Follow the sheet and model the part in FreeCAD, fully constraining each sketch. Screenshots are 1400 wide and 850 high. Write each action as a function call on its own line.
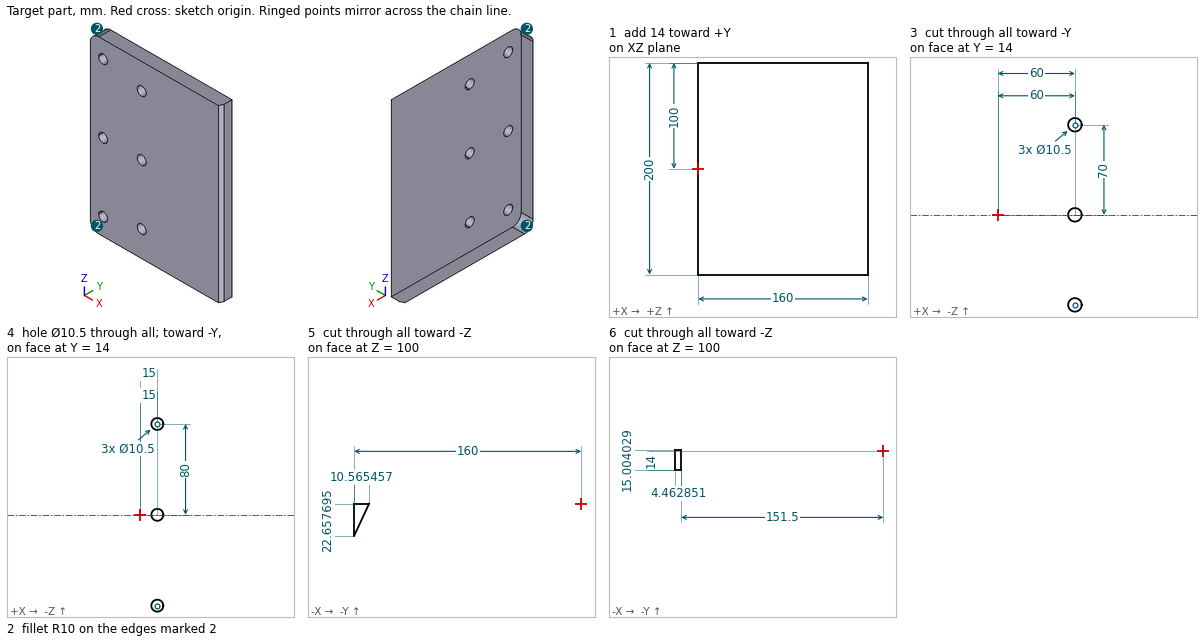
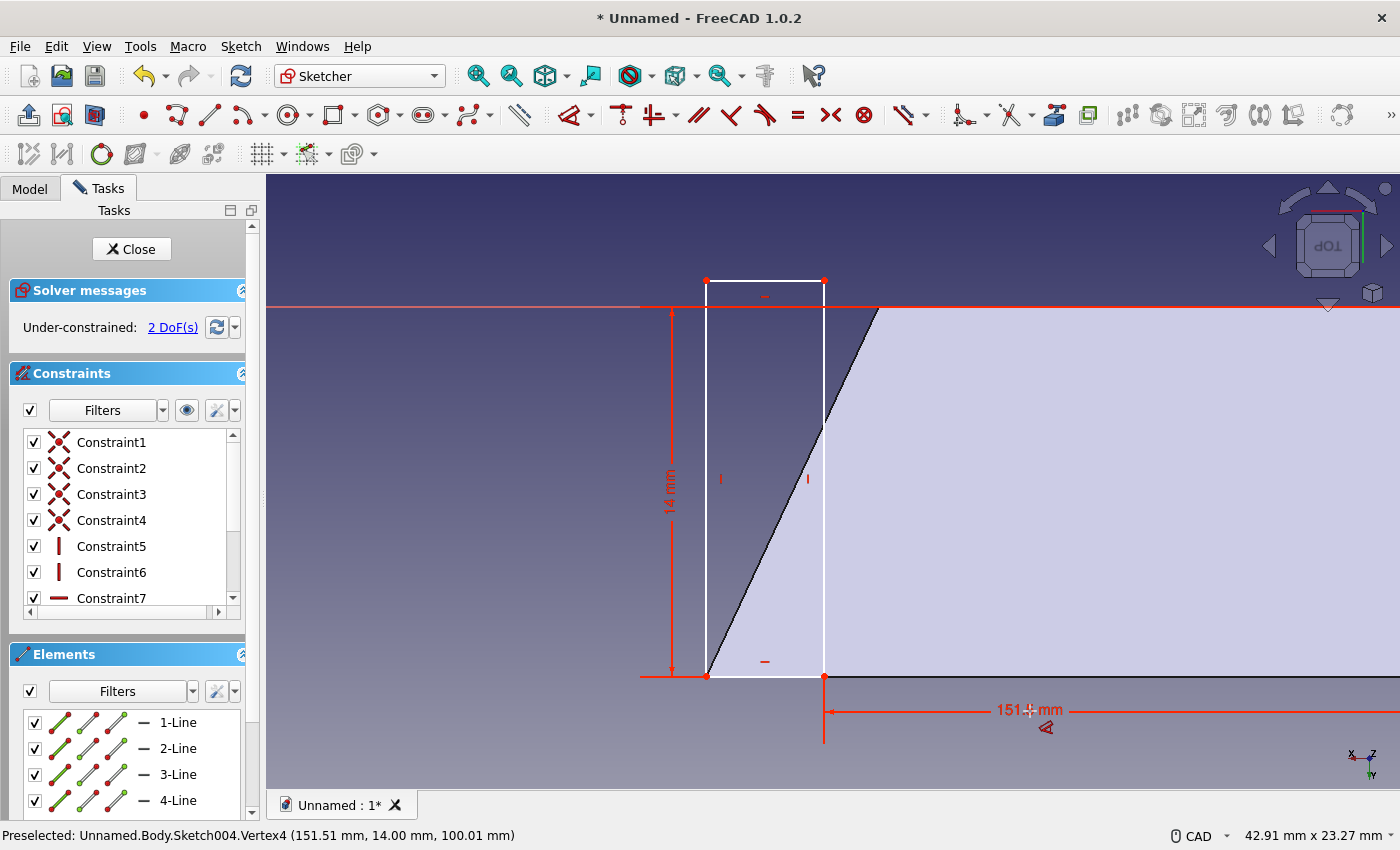
click(741, 677)
click(765, 711)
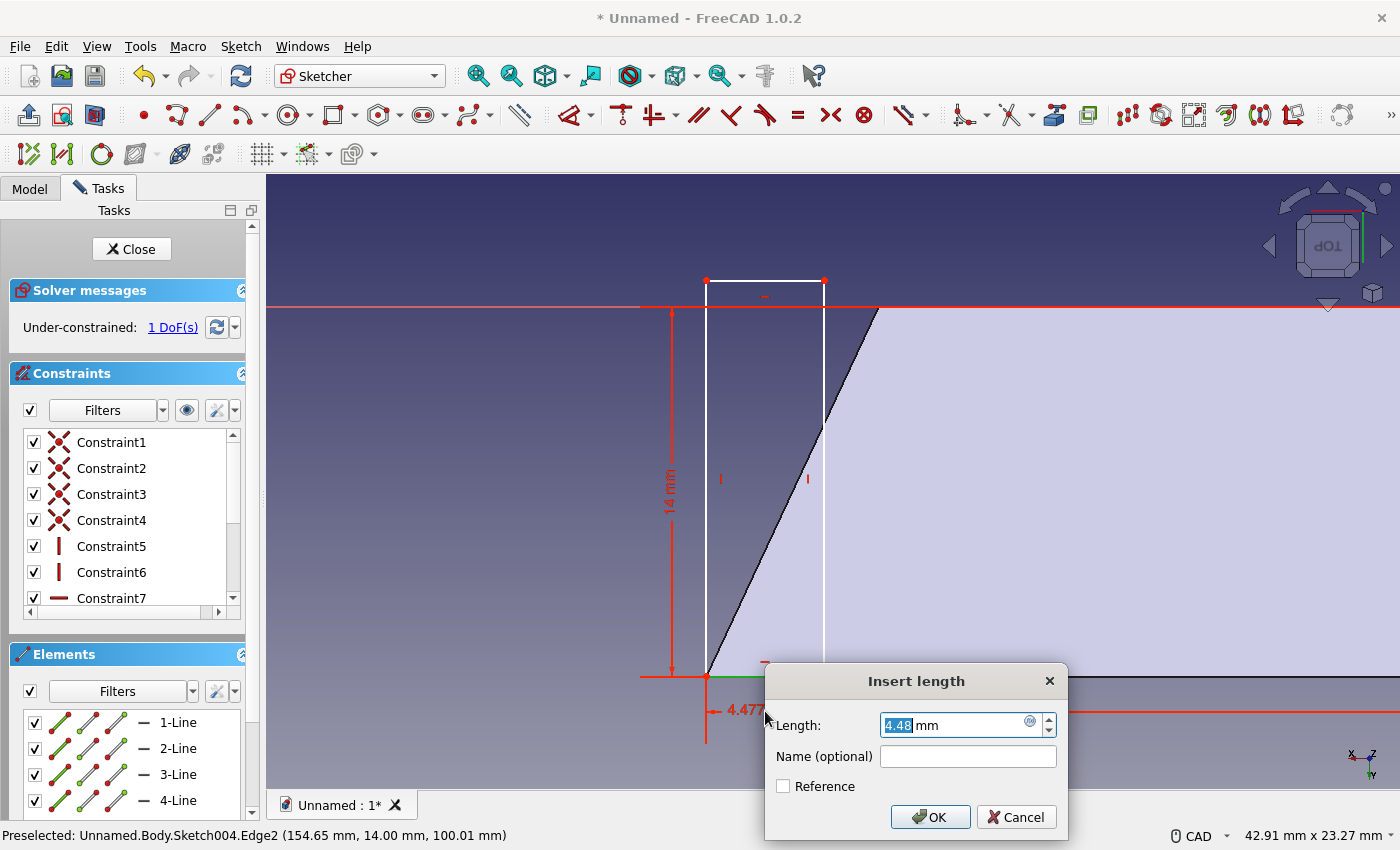
text(4.462851)
key(Return)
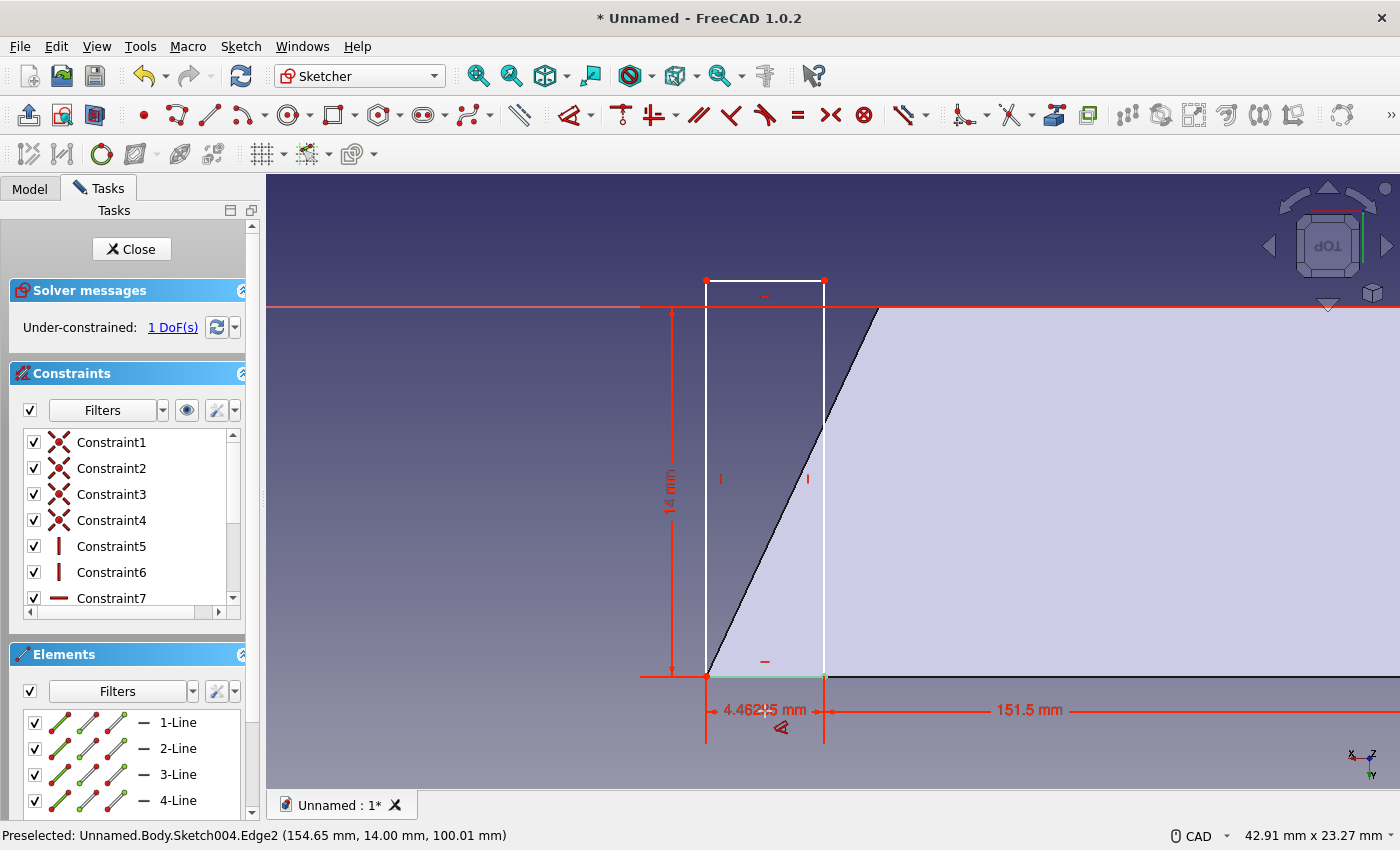
click(706, 400)
click(672, 388)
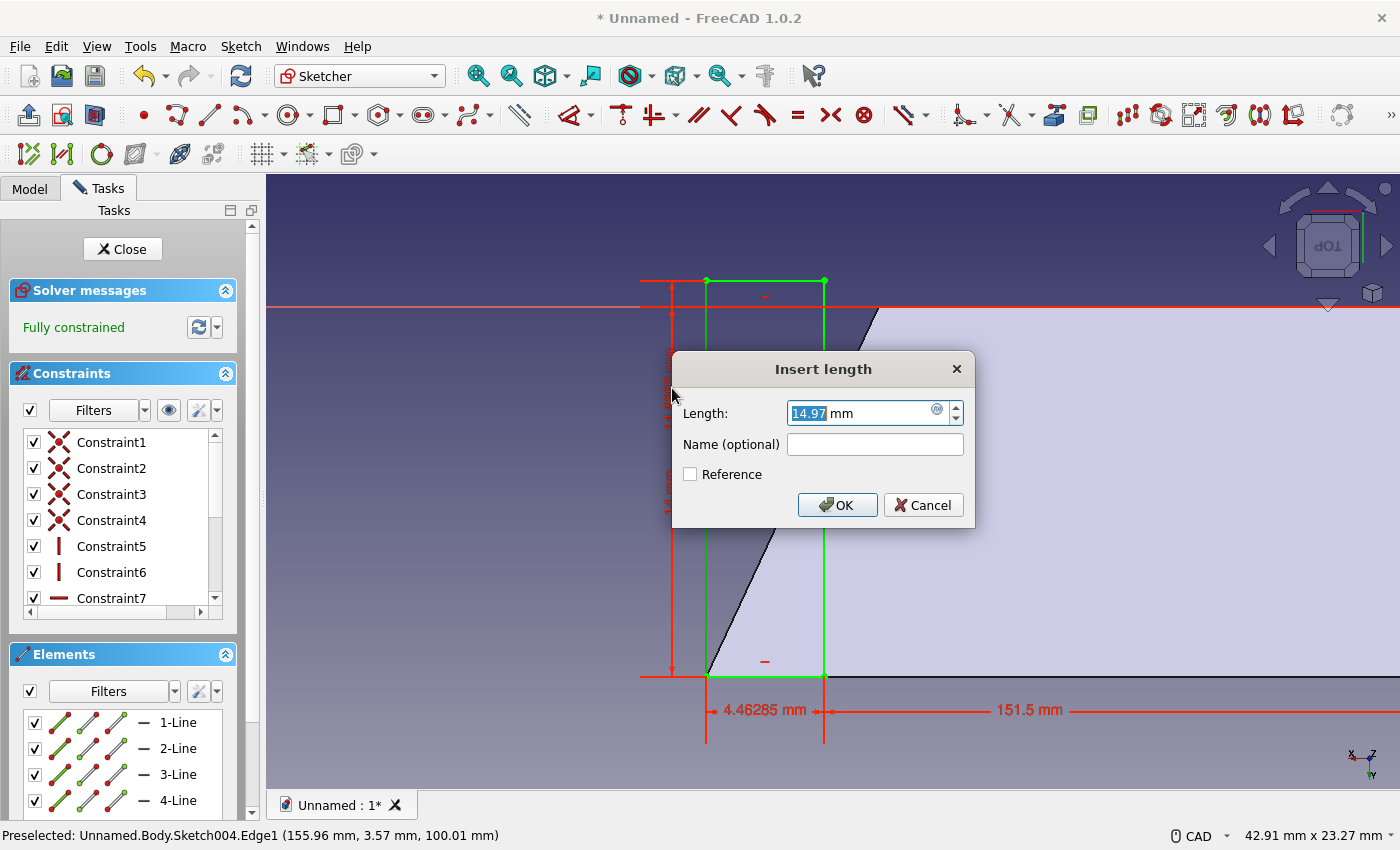
text(15.004029)
key(Return)
key(Escape)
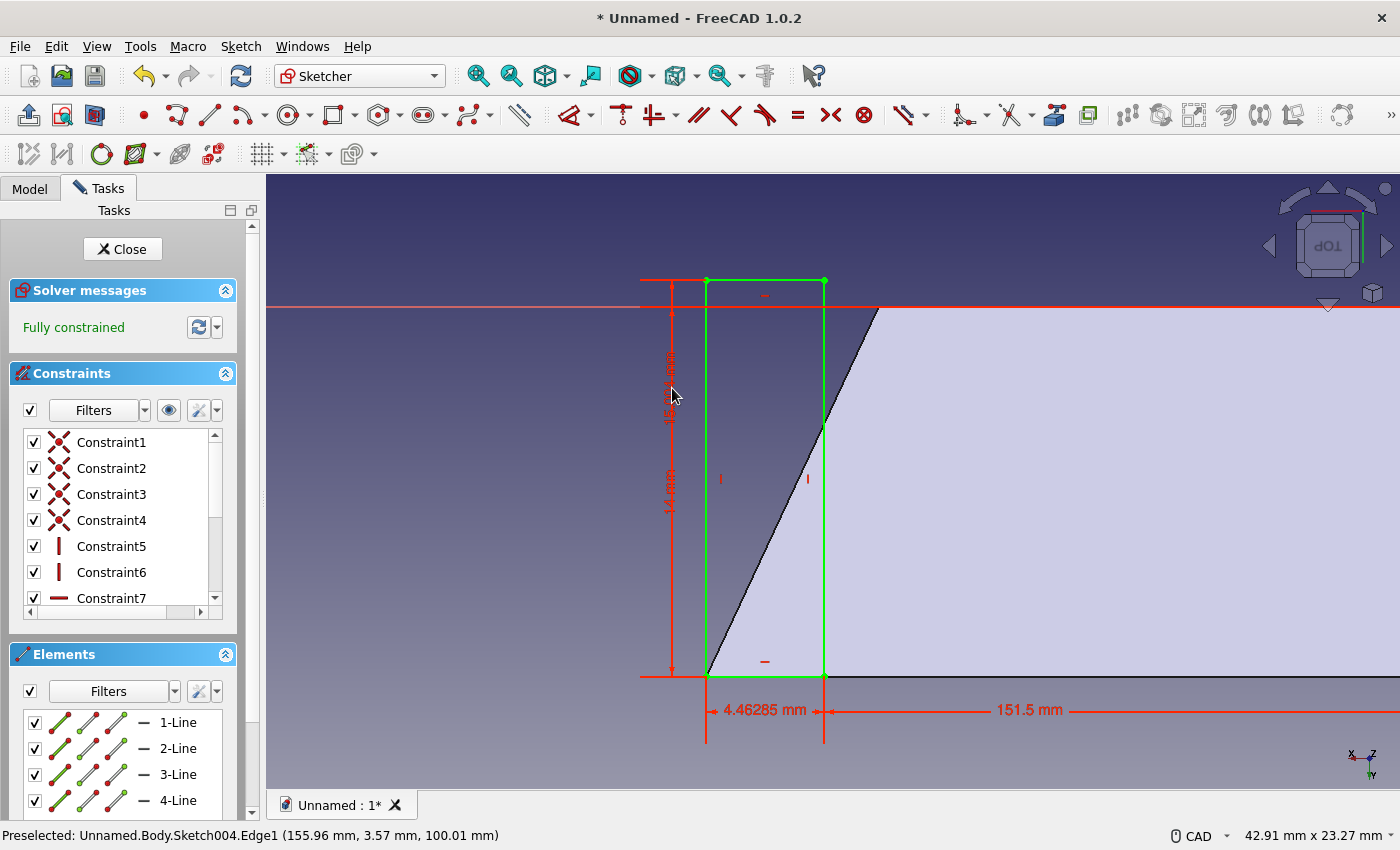
click(123, 249)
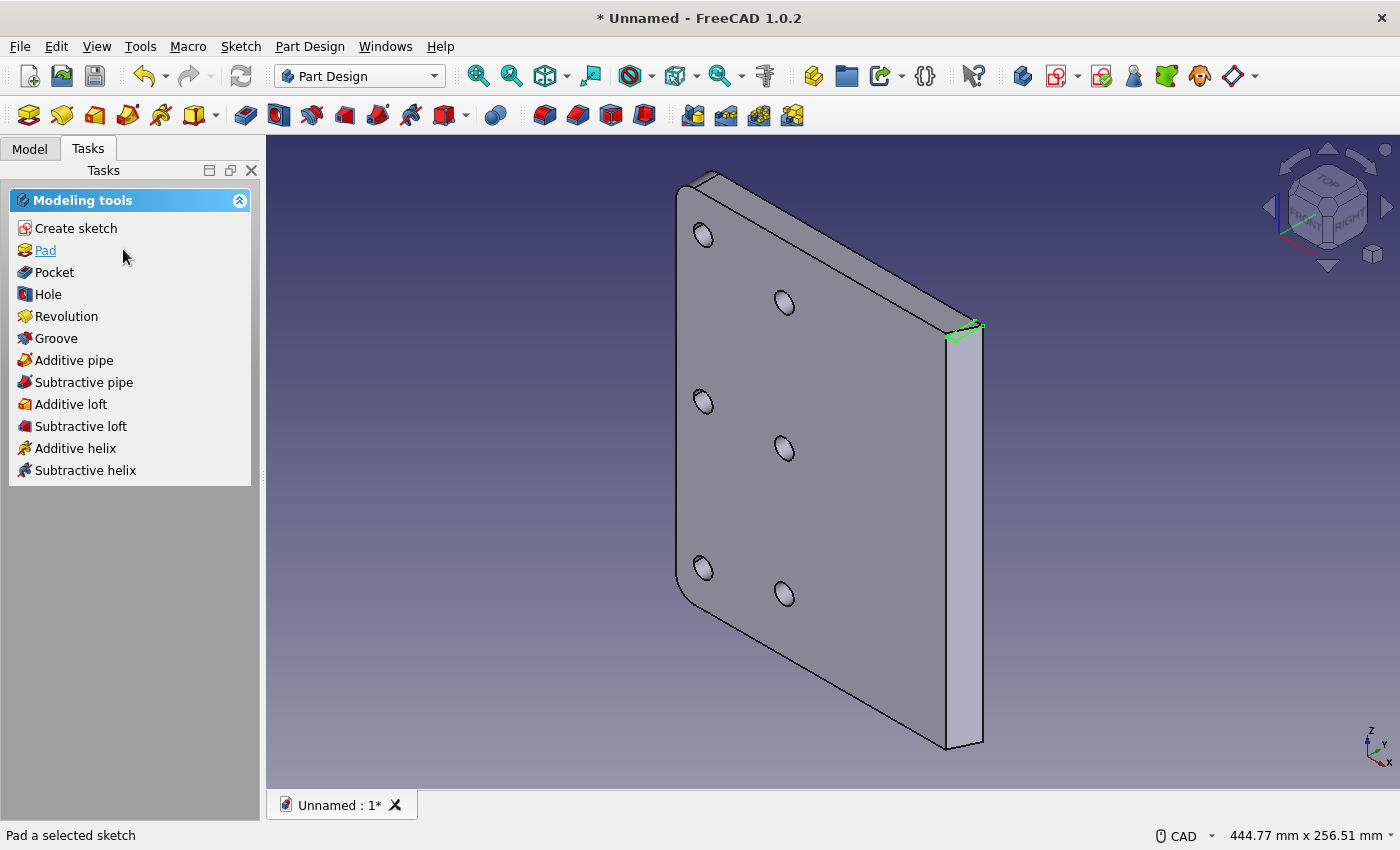
click(246, 116)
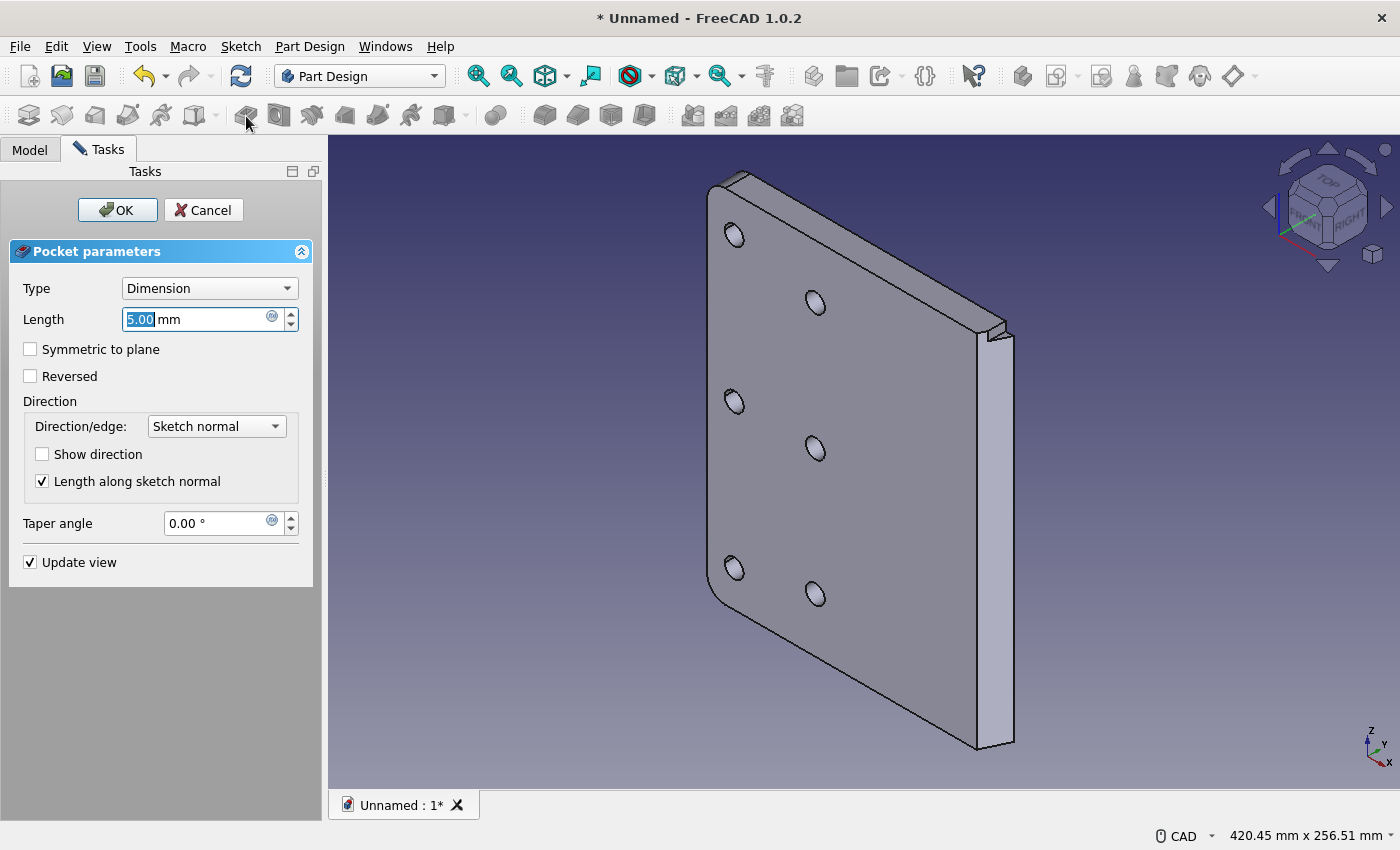
click(210, 288)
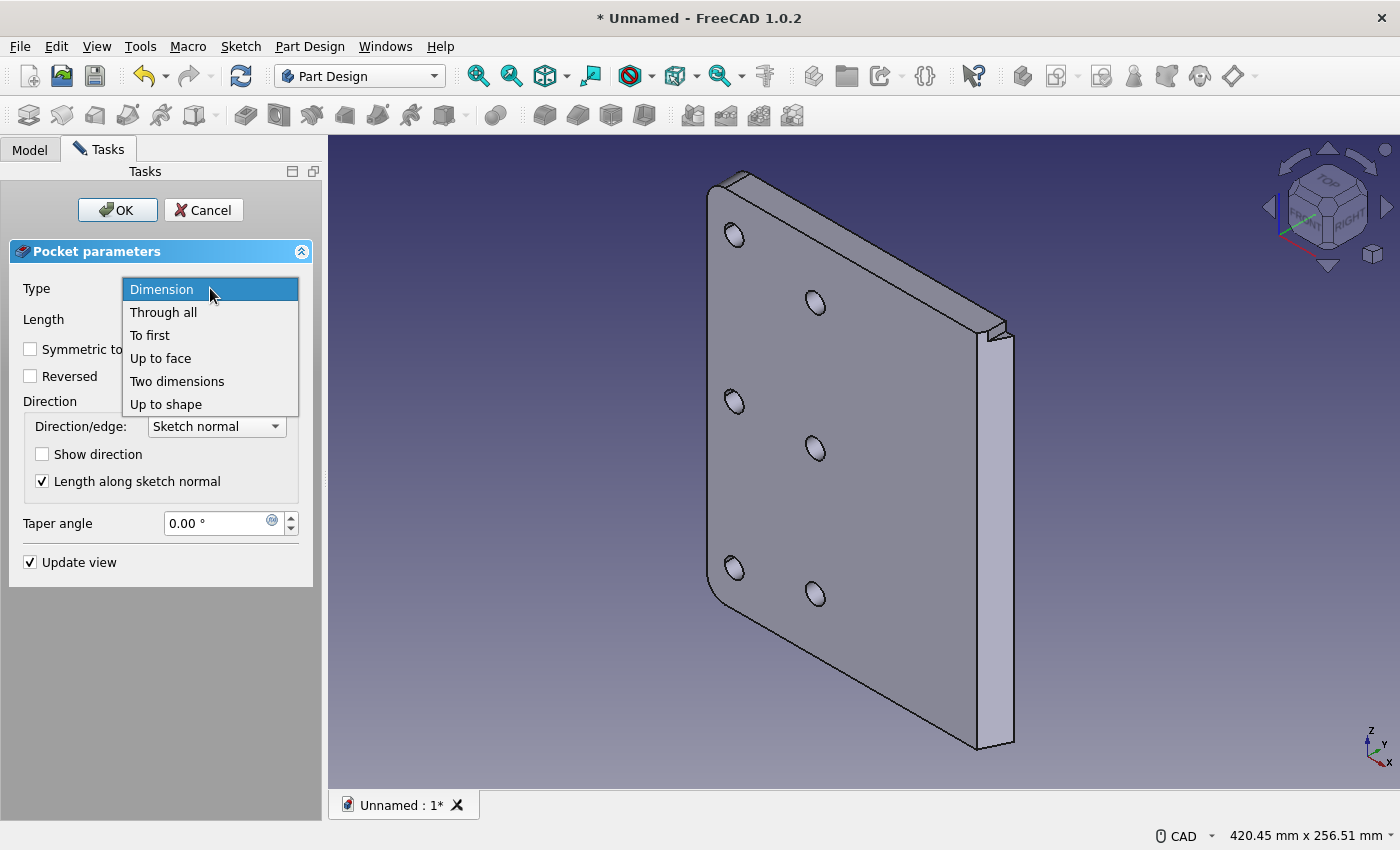
click(208, 312)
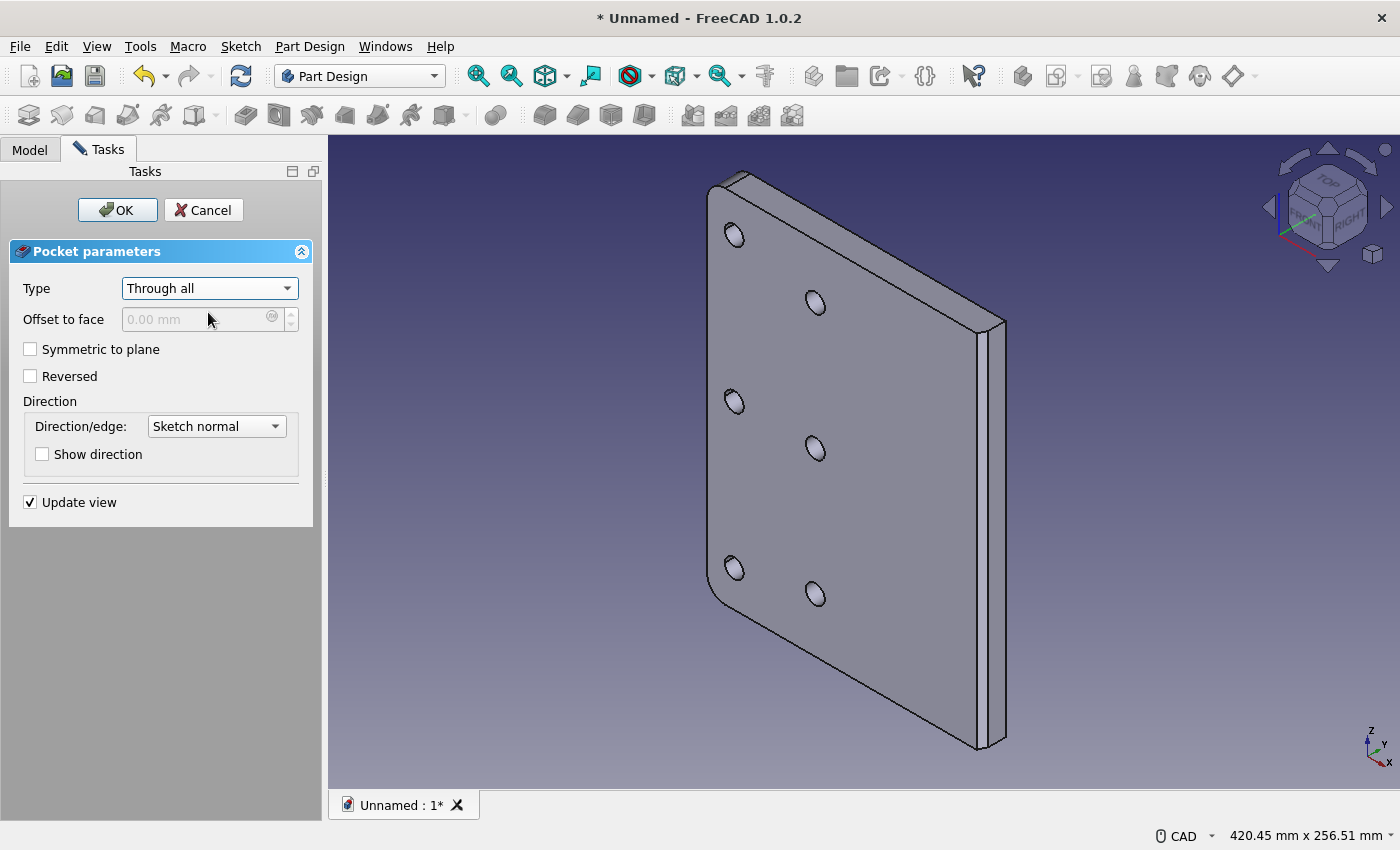
click(118, 210)